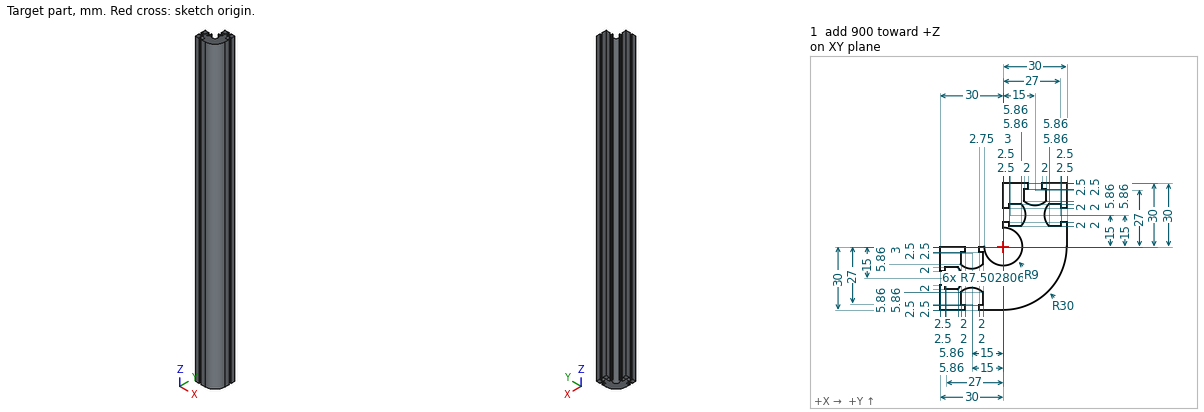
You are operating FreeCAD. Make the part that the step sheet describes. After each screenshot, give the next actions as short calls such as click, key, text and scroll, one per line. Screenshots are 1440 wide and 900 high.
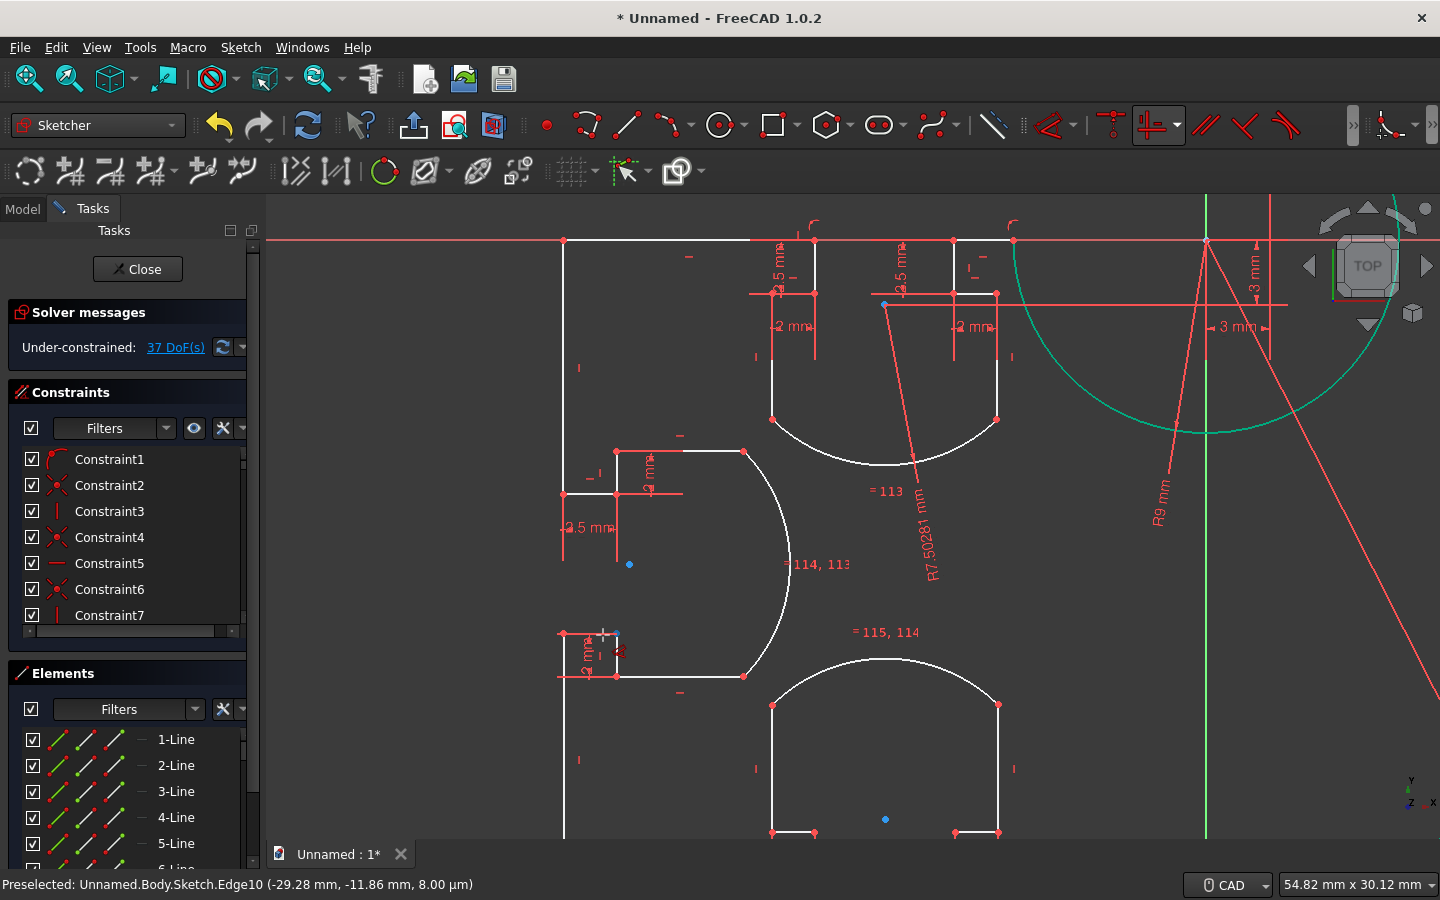
click(601, 634)
click(590, 600)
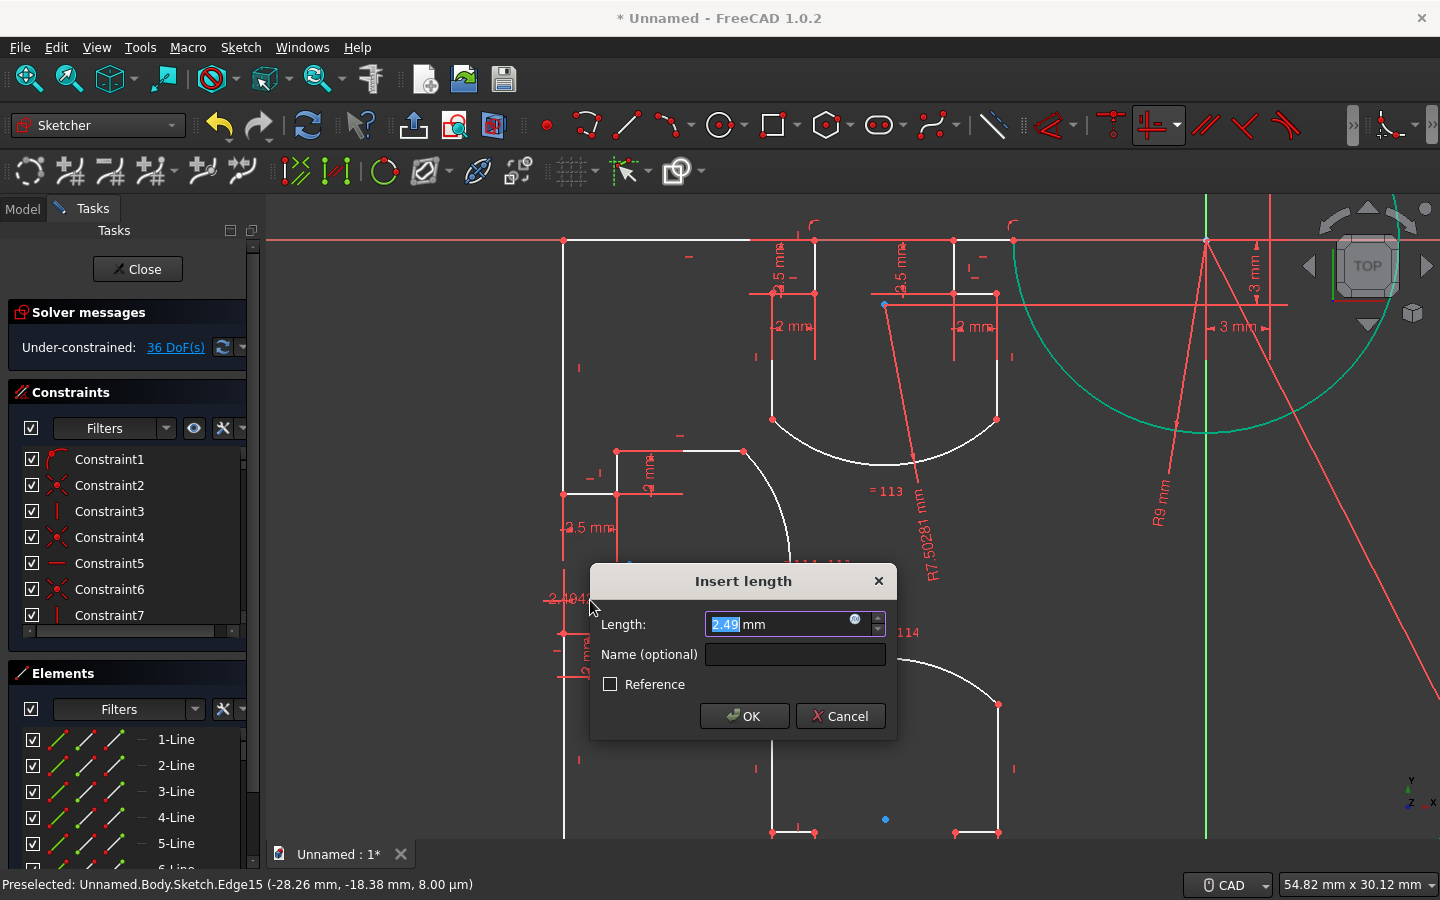
text(2.5)
key(Return)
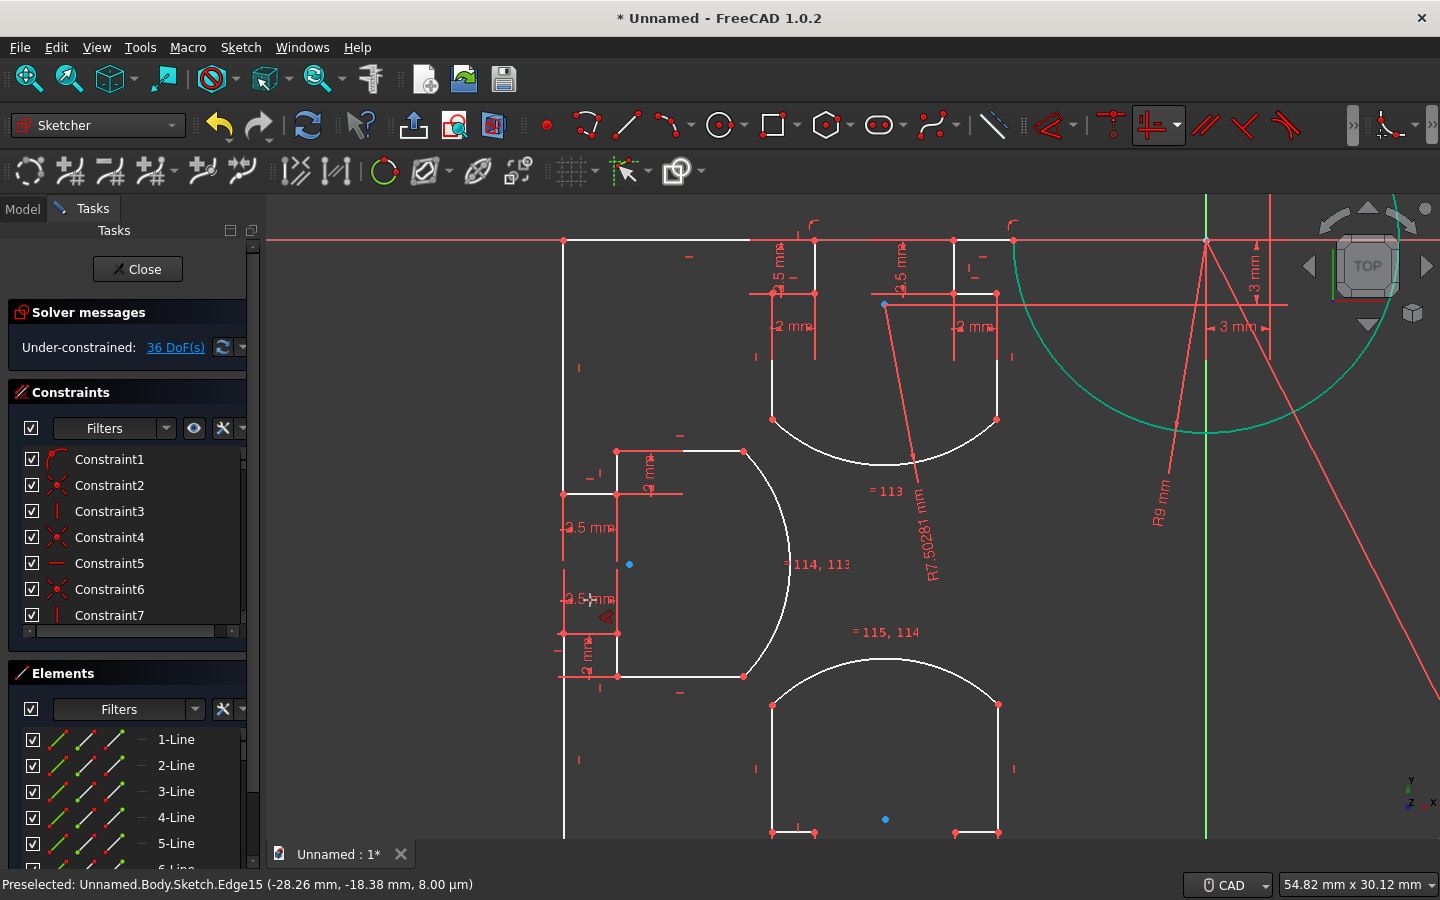
scroll(603, 636, down, 6)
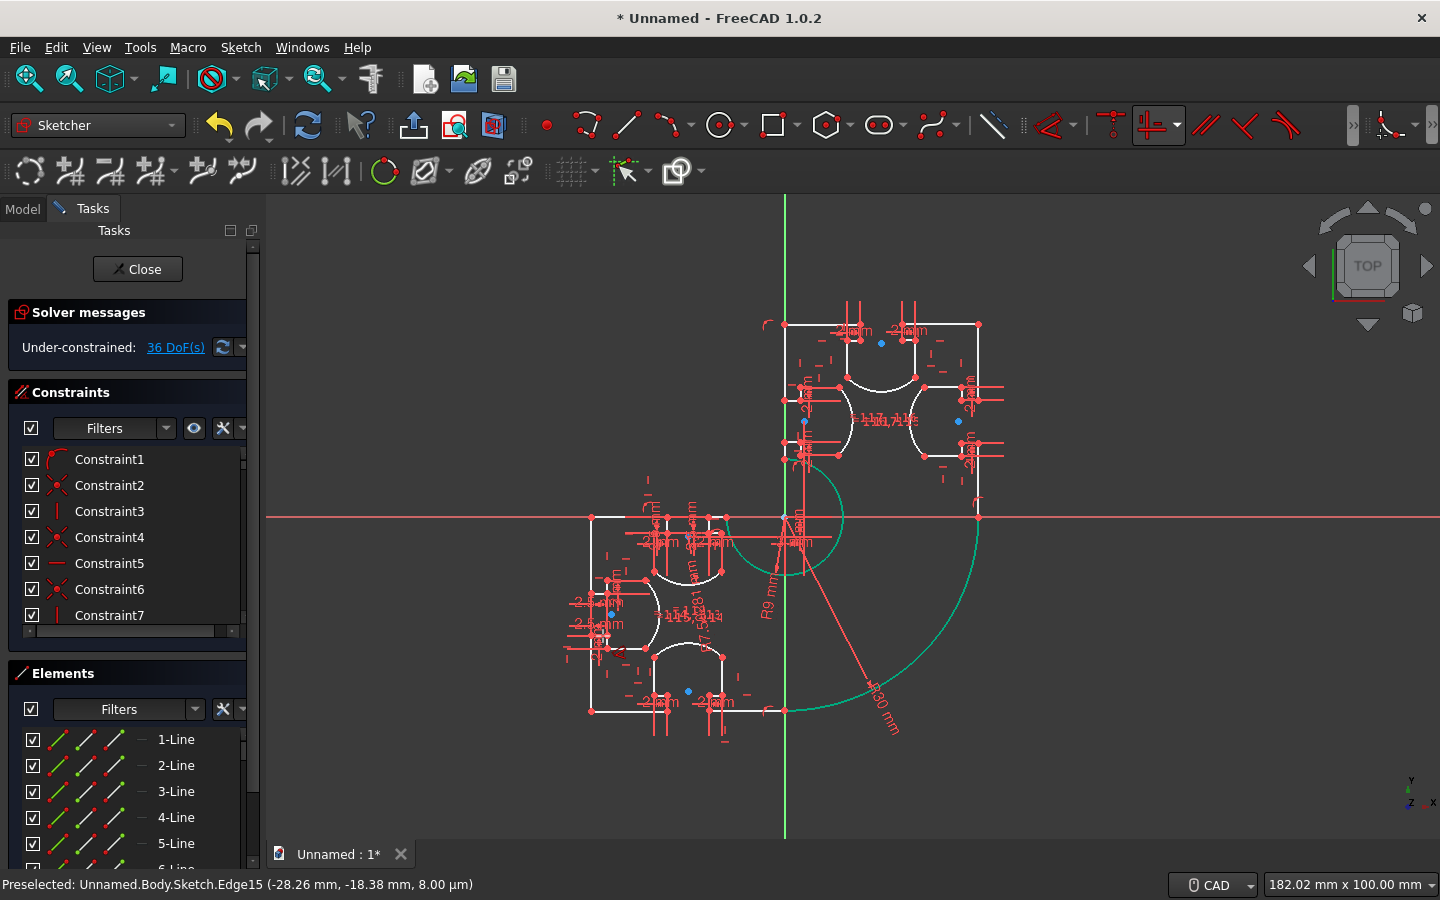
scroll(667, 707, up, 6)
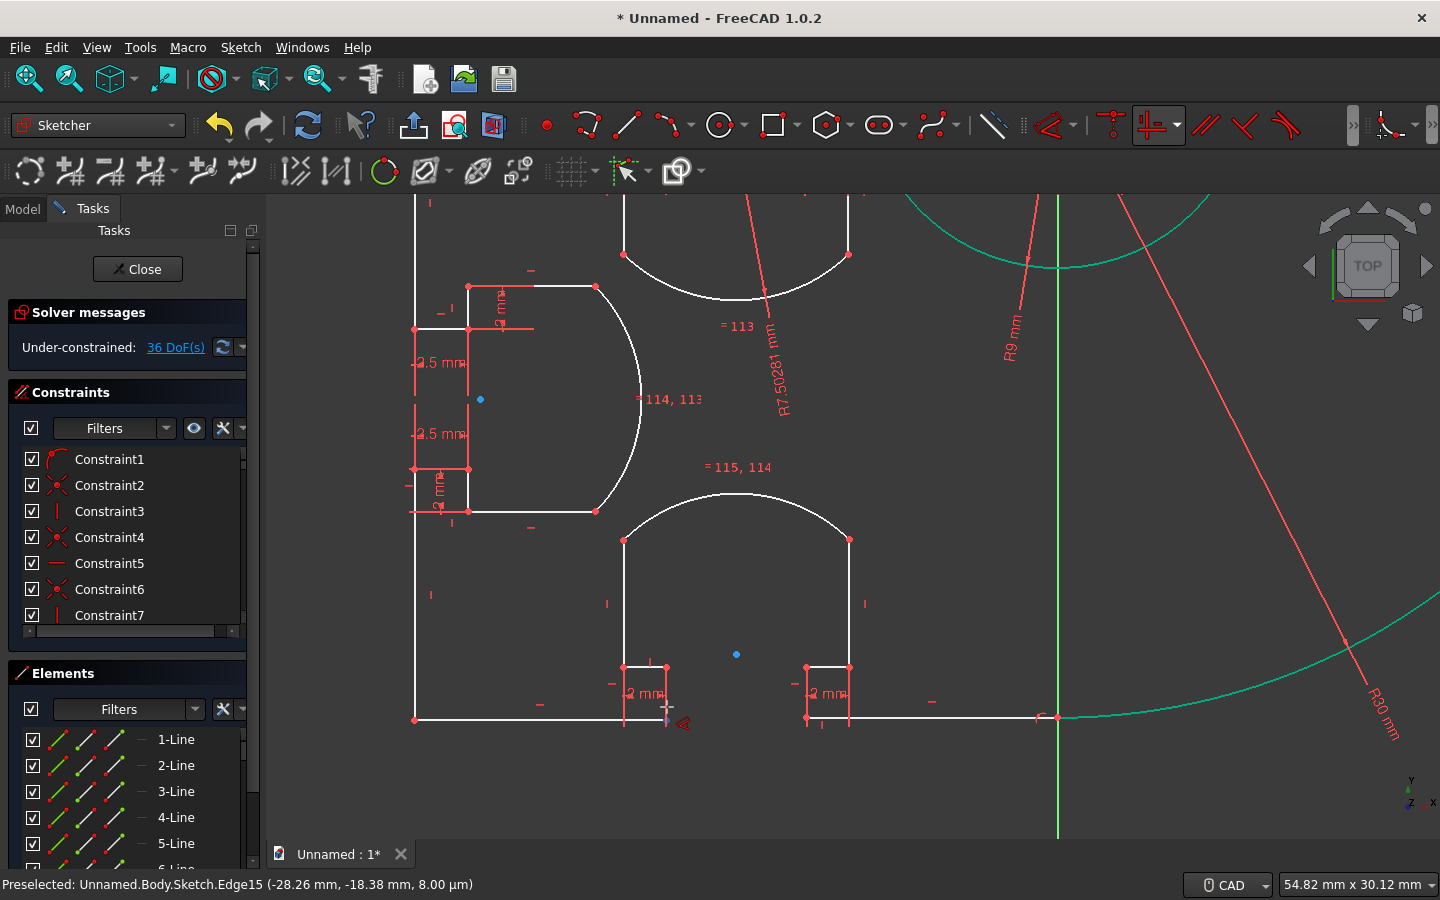
click(666, 704)
click(724, 694)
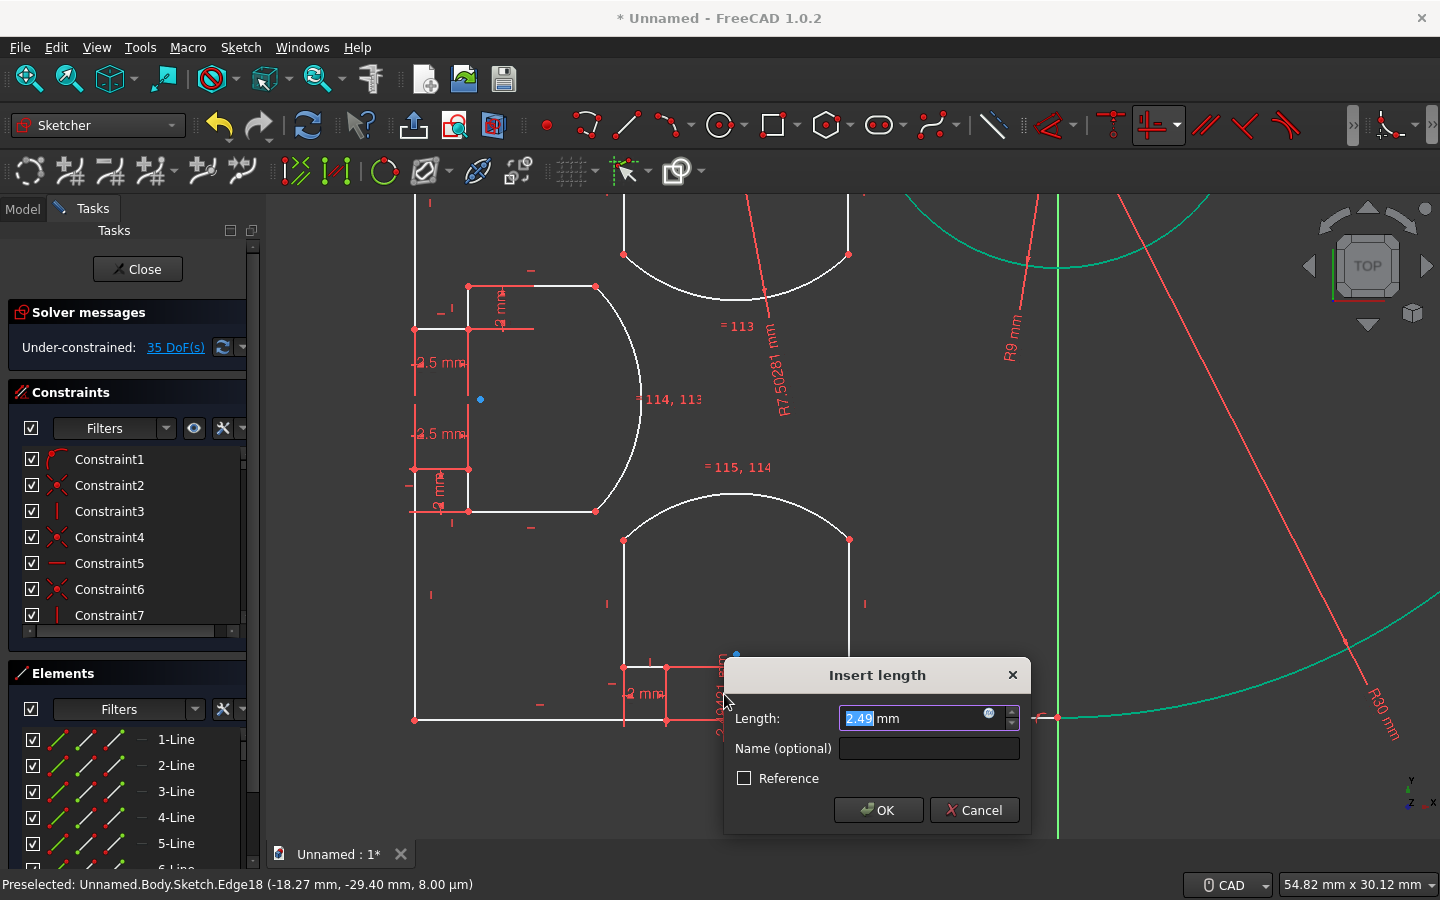
text(2.5)
key(Return)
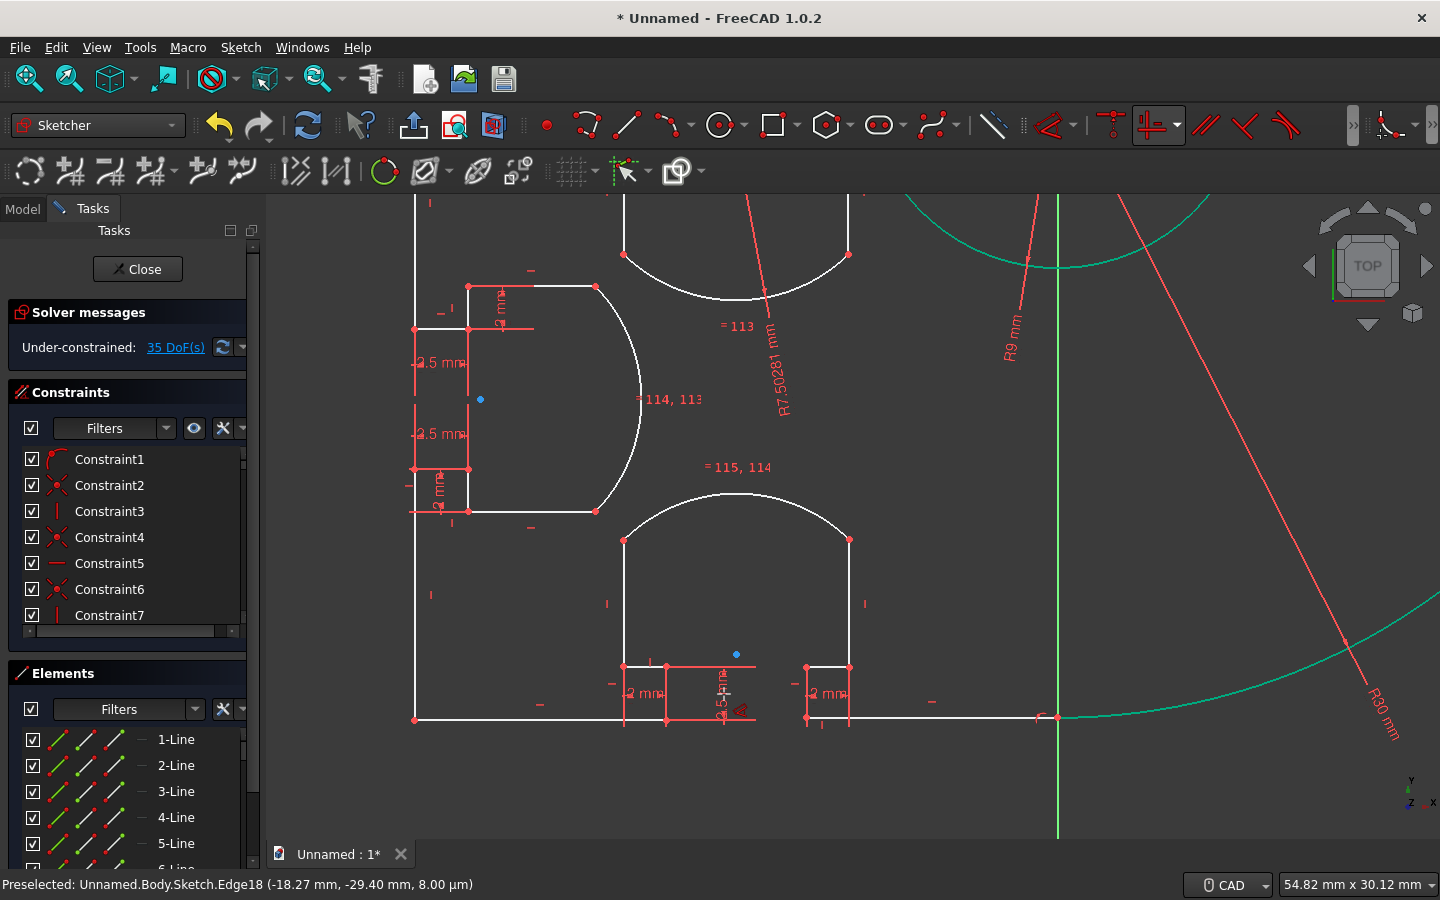
click(807, 682)
click(865, 675)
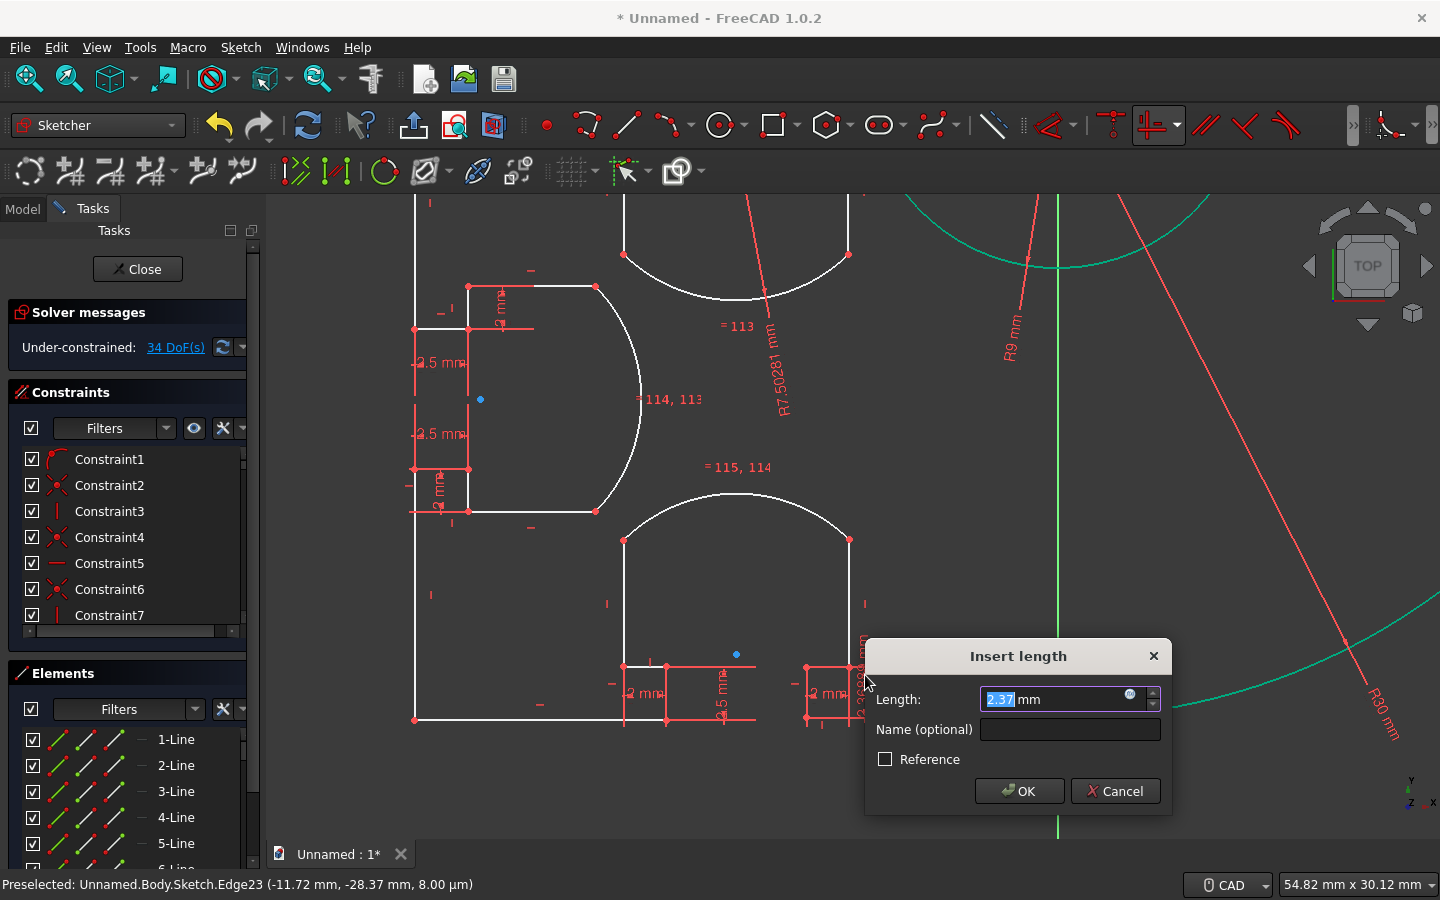
text(2.5)
key(Return)